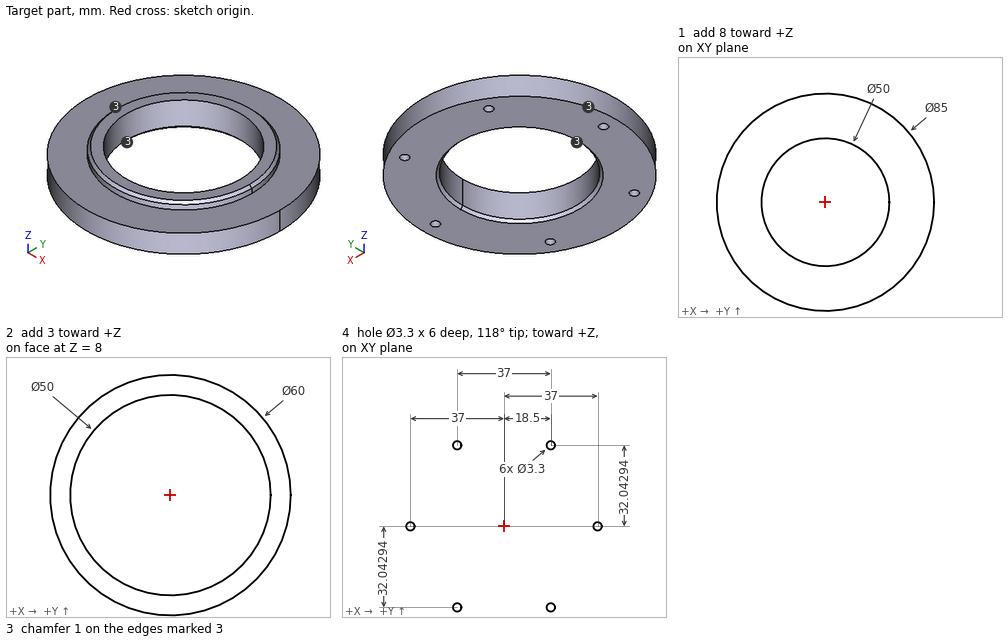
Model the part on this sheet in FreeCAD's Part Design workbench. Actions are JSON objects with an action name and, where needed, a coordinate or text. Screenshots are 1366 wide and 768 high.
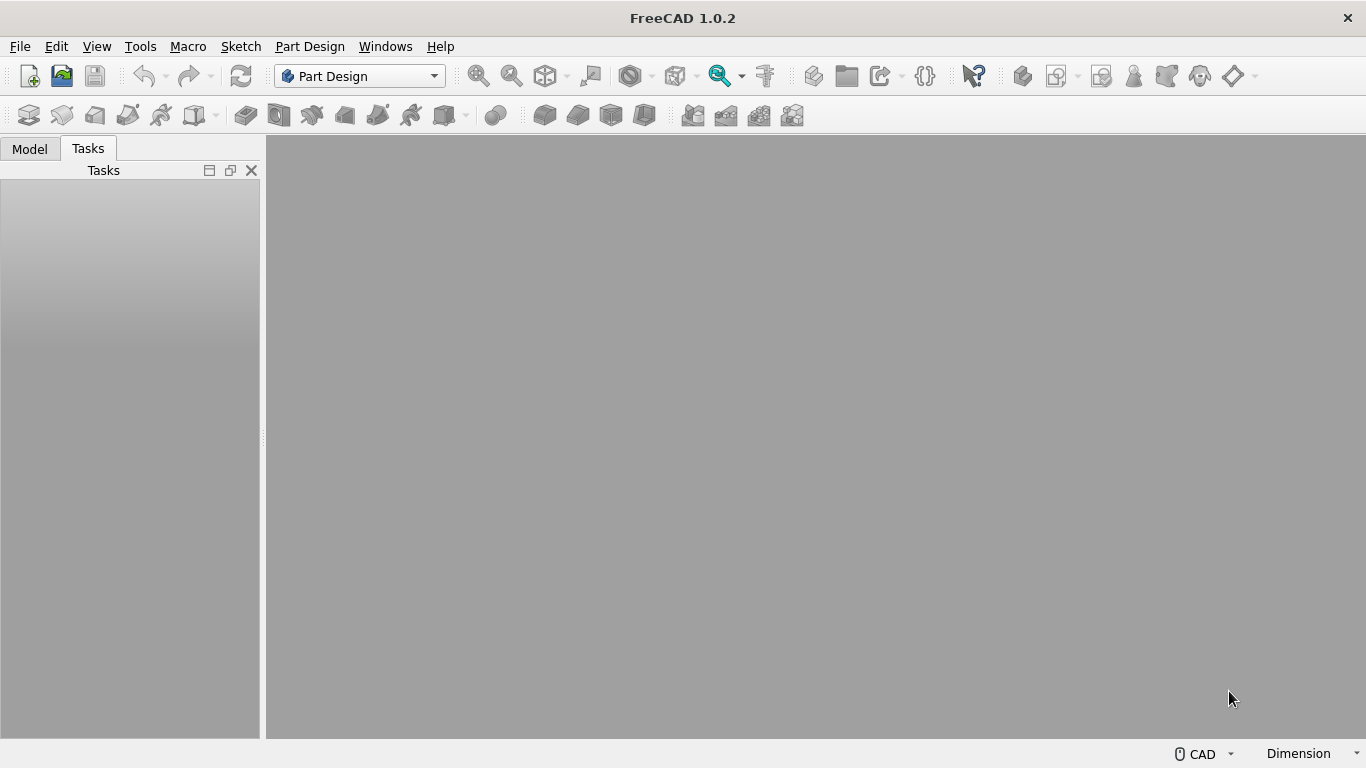
{"action": "left_click", "coordinate": [29, 76]}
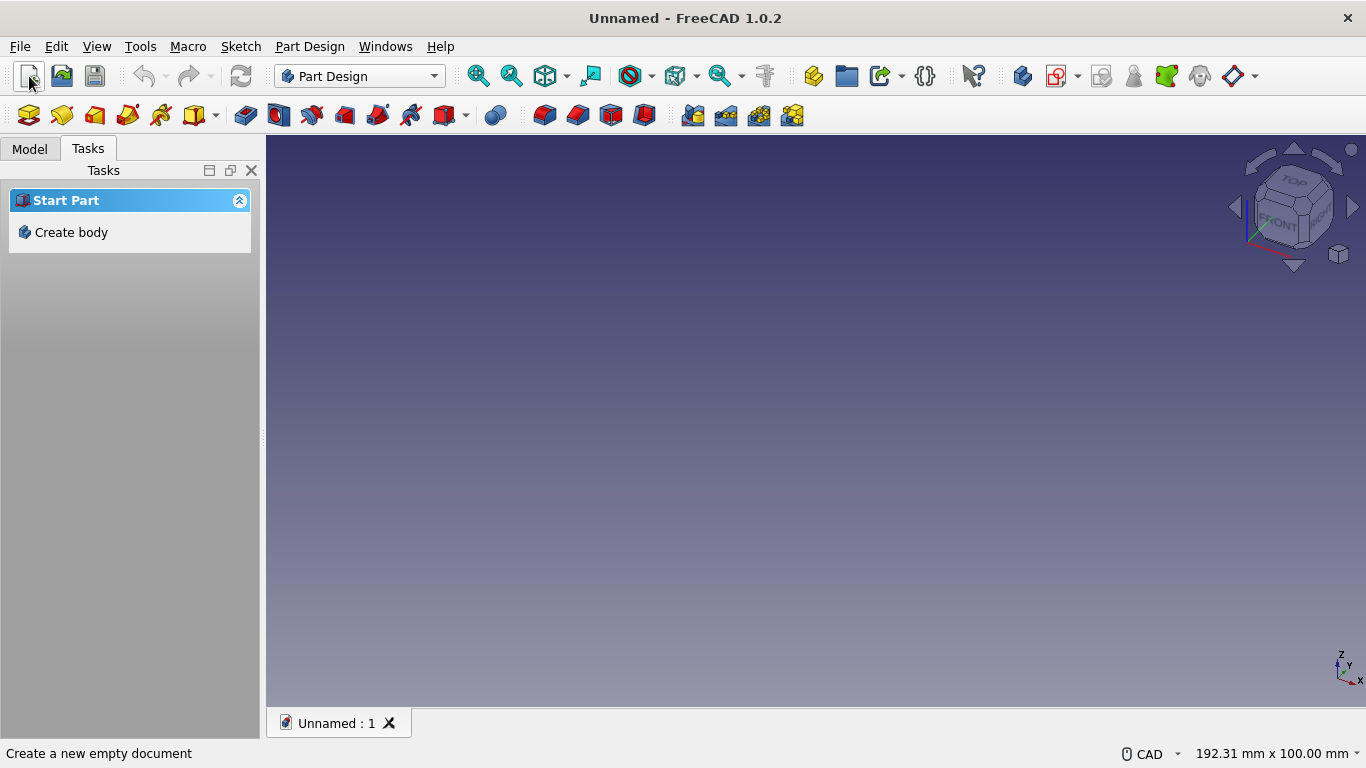
{"action": "left_click", "coordinate": [1056, 76]}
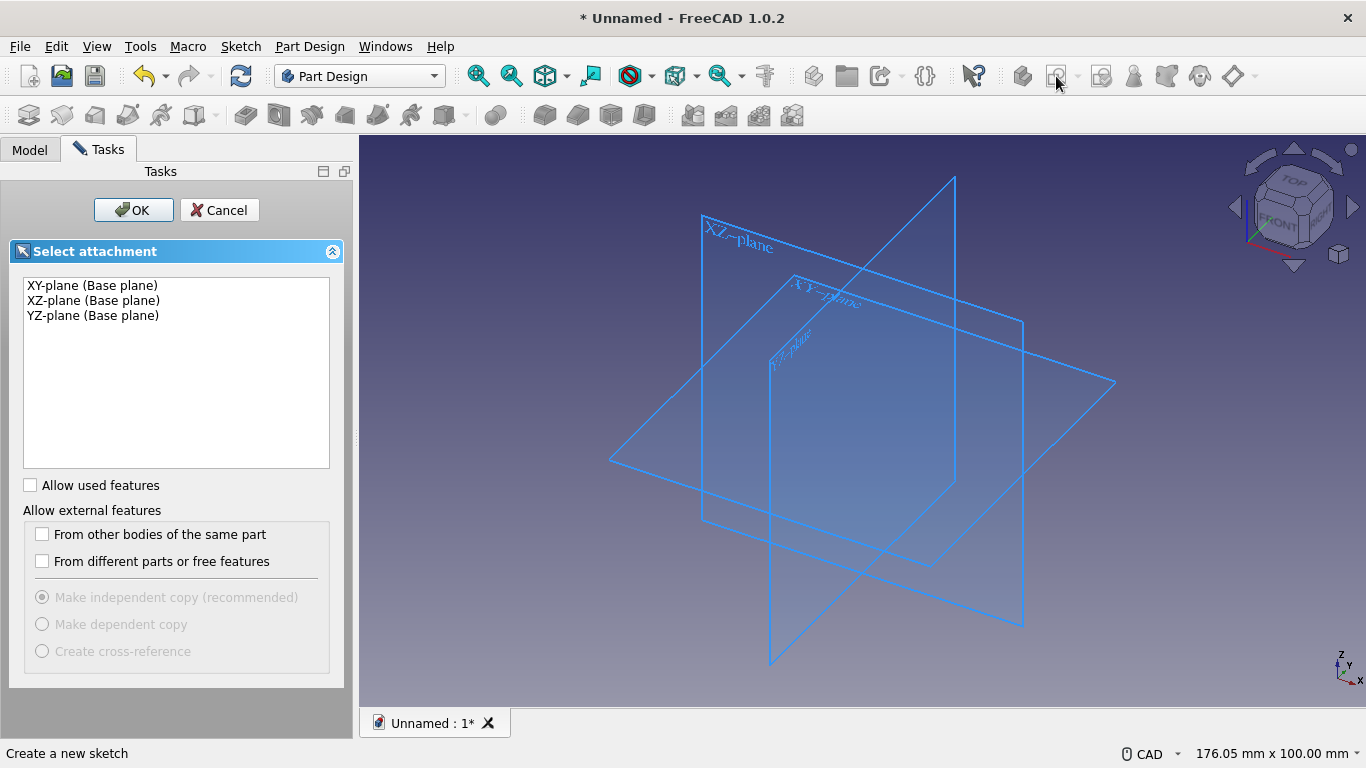
{"action": "left_click", "coordinate": [84, 286]}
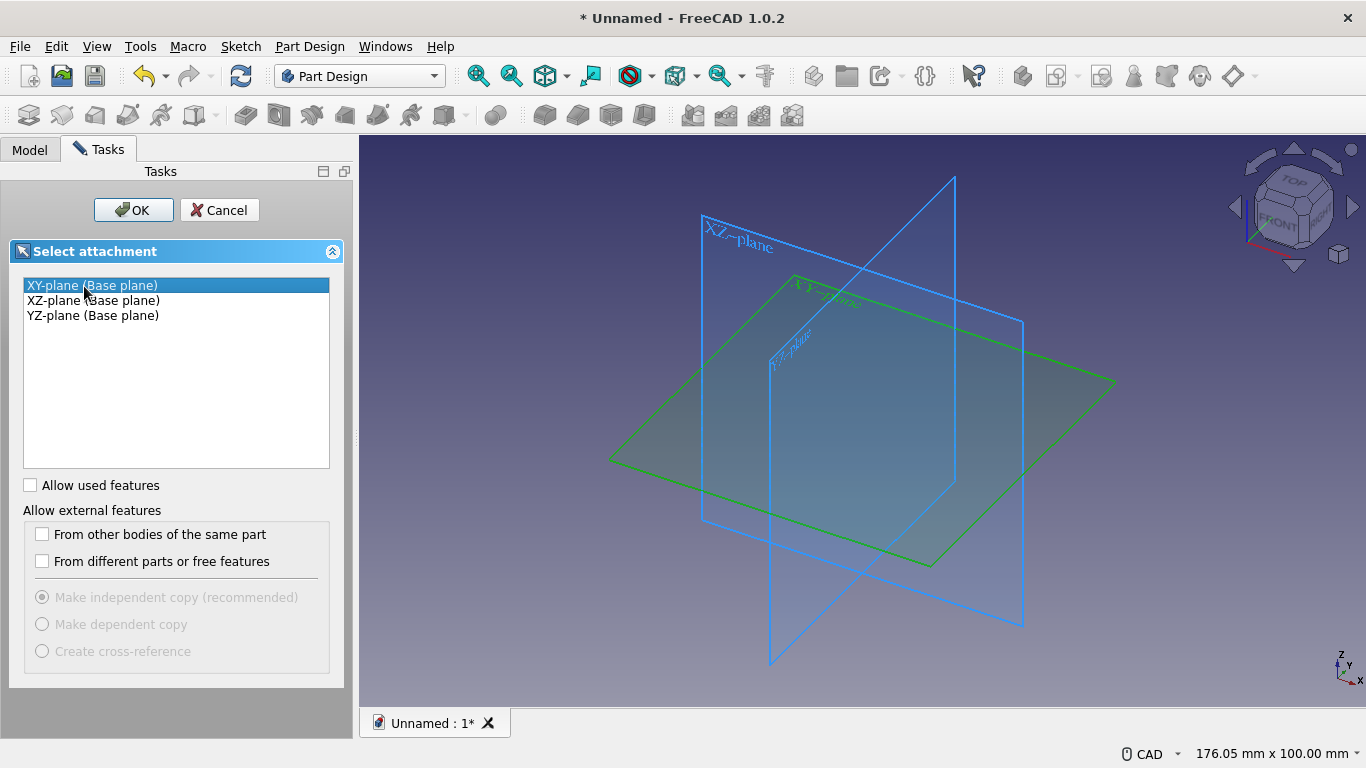
{"action": "left_click", "coordinate": [134, 210]}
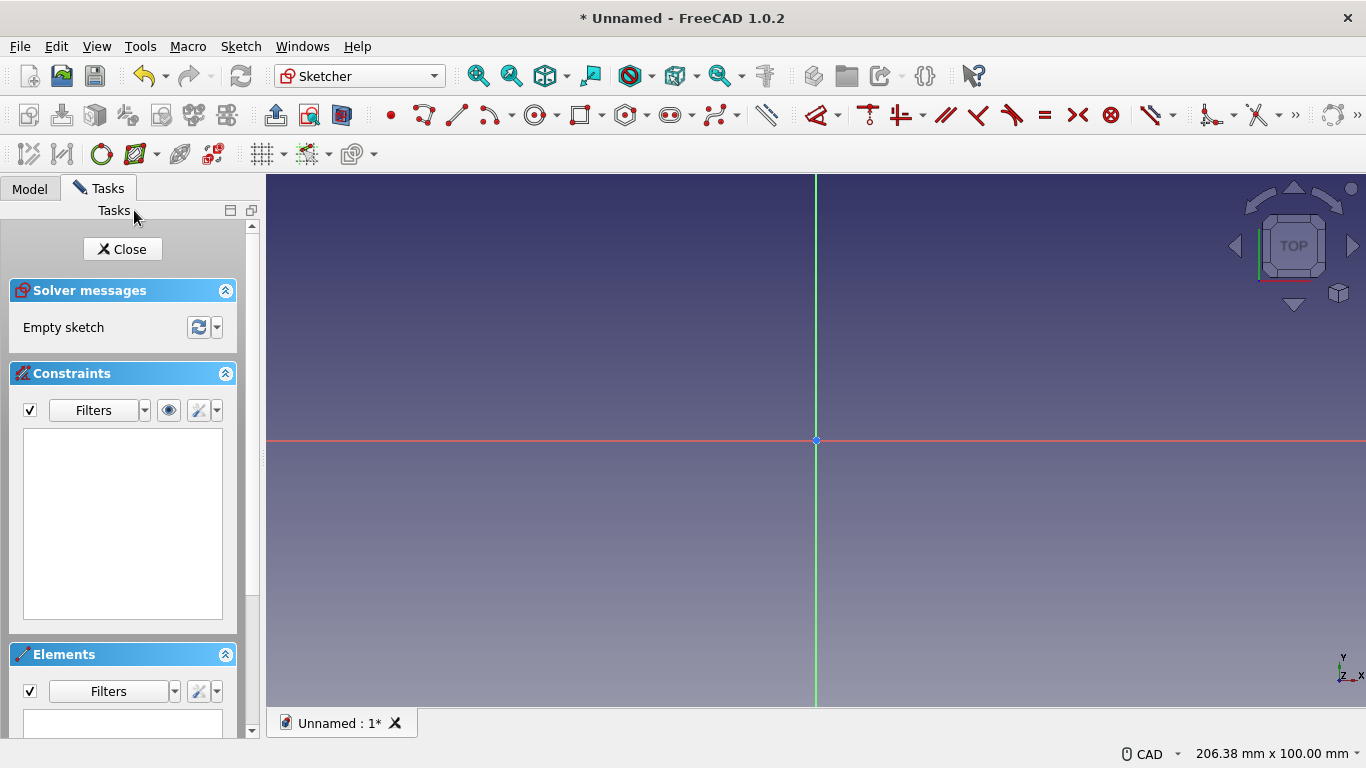
{"action": "scroll", "coordinate": [438, 440], "scroll_direction": "down", "scroll_amount": 1}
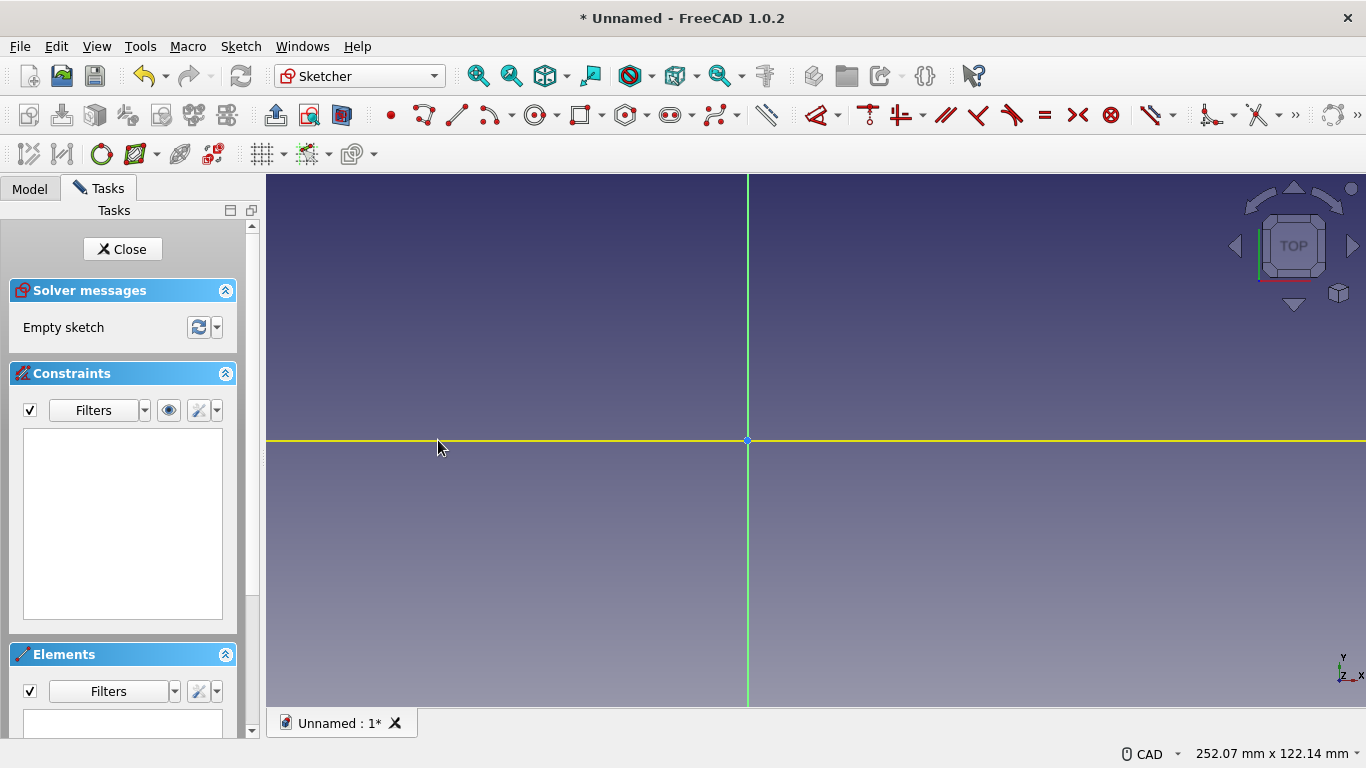
{"action": "left_click", "coordinate": [534, 116]}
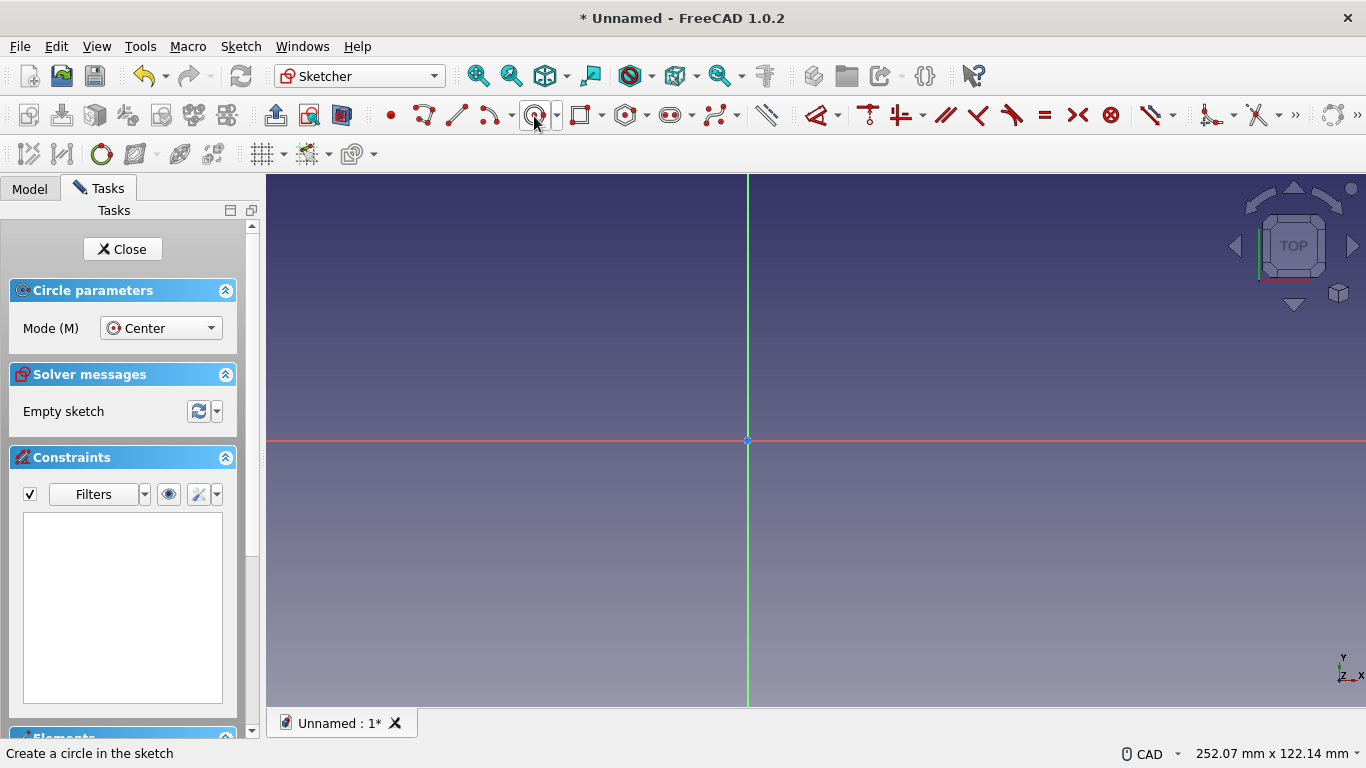
{"action": "left_click", "coordinate": [748, 440]}
{"action": "mouse_move", "coordinate": [879, 309]}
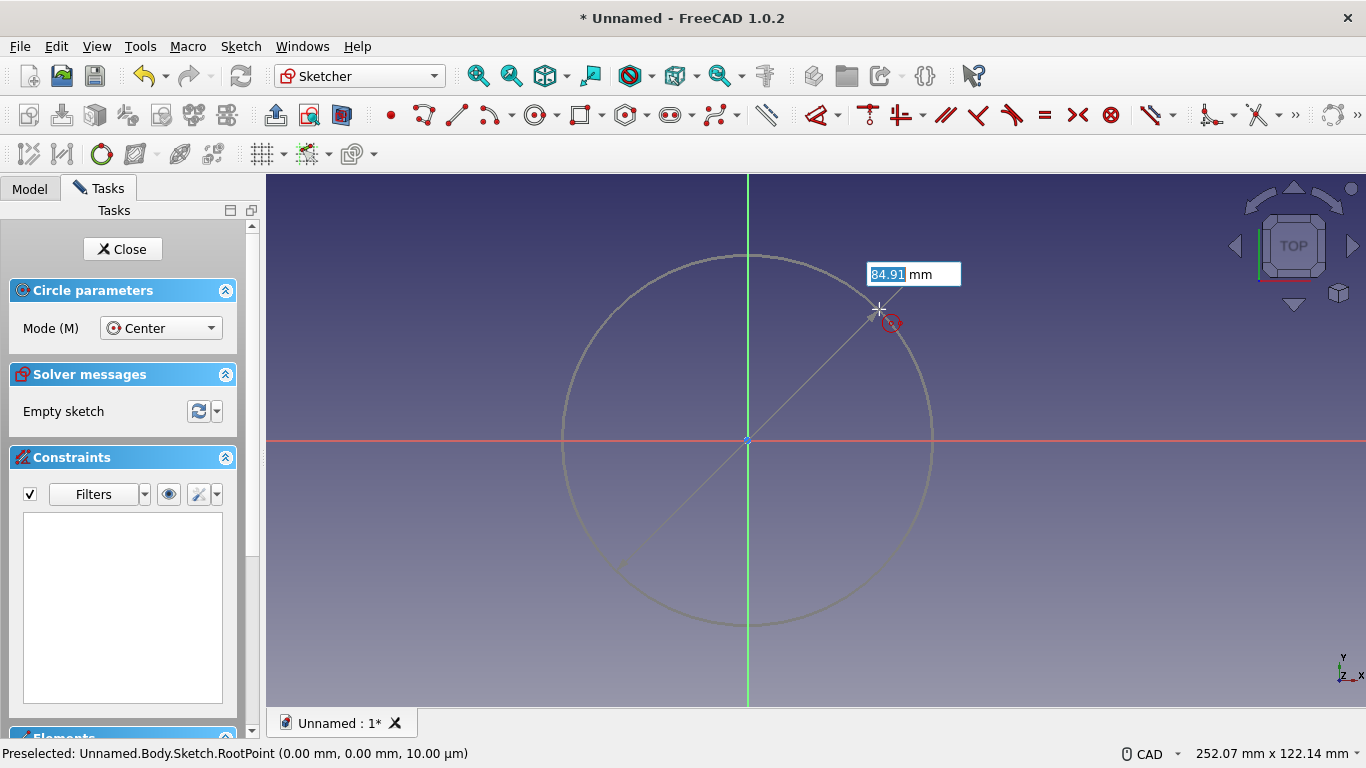
{"action": "type", "text": "85"}
{"action": "key", "text": "Return"}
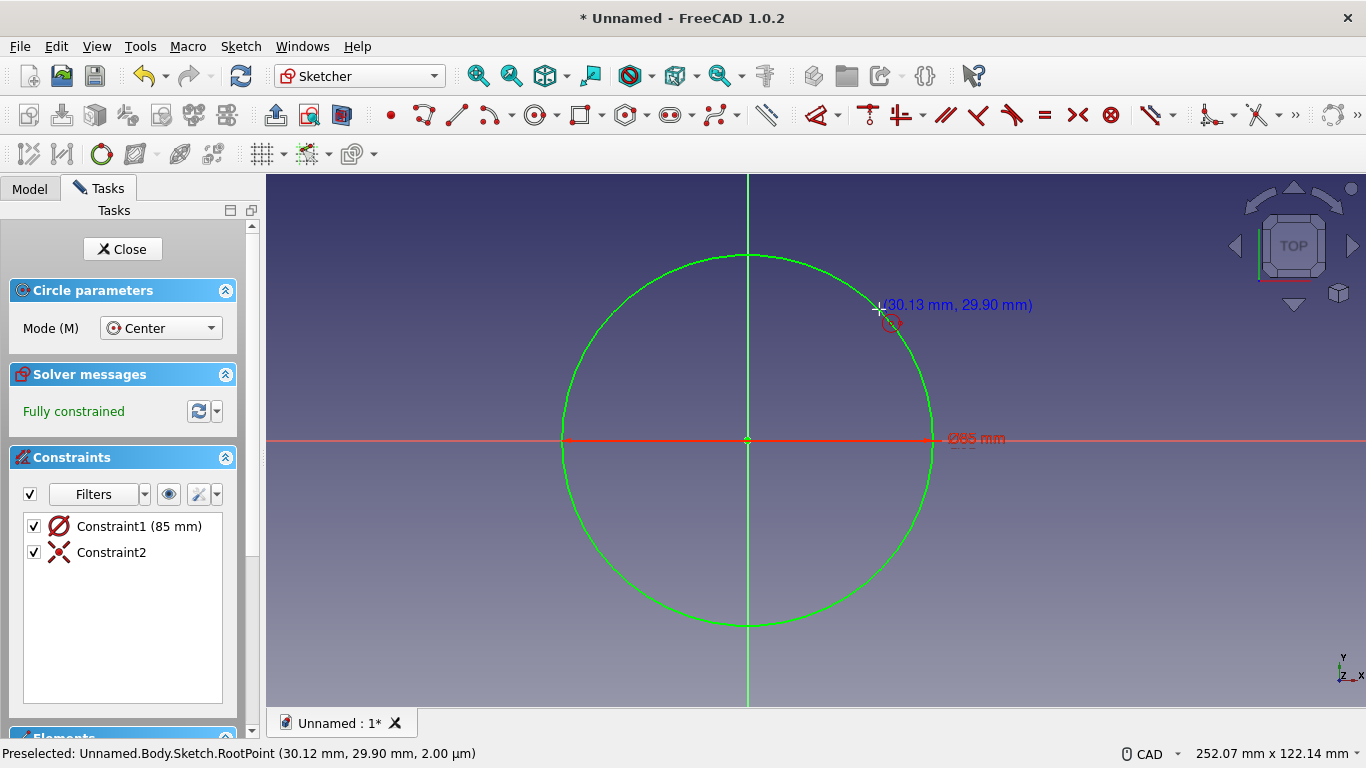
{"action": "left_click", "coordinate": [748, 440]}
{"action": "mouse_move", "coordinate": [825, 363]}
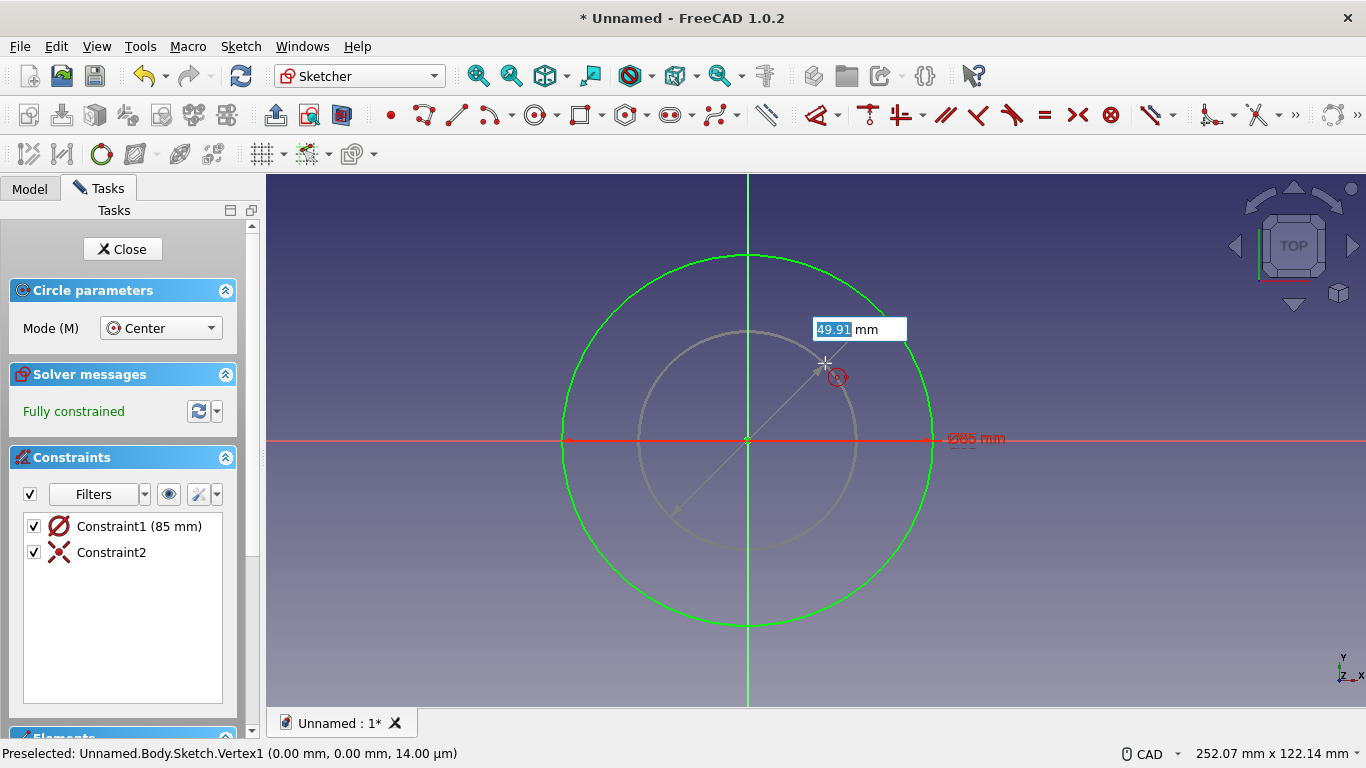
{"action": "type", "text": "50"}
{"action": "key", "text": "Return"}
{"action": "key", "text": "Escape"}